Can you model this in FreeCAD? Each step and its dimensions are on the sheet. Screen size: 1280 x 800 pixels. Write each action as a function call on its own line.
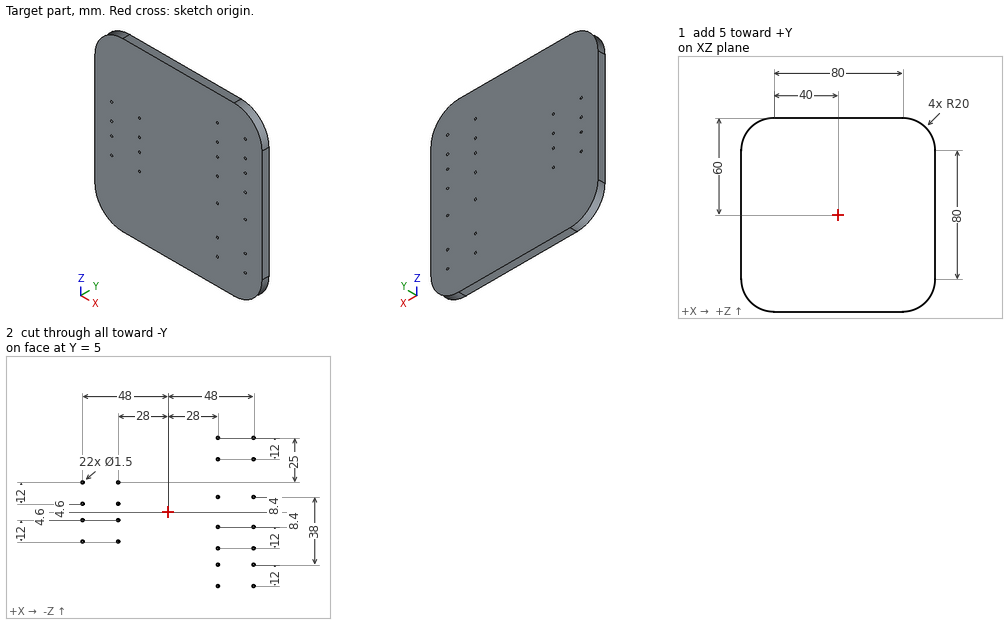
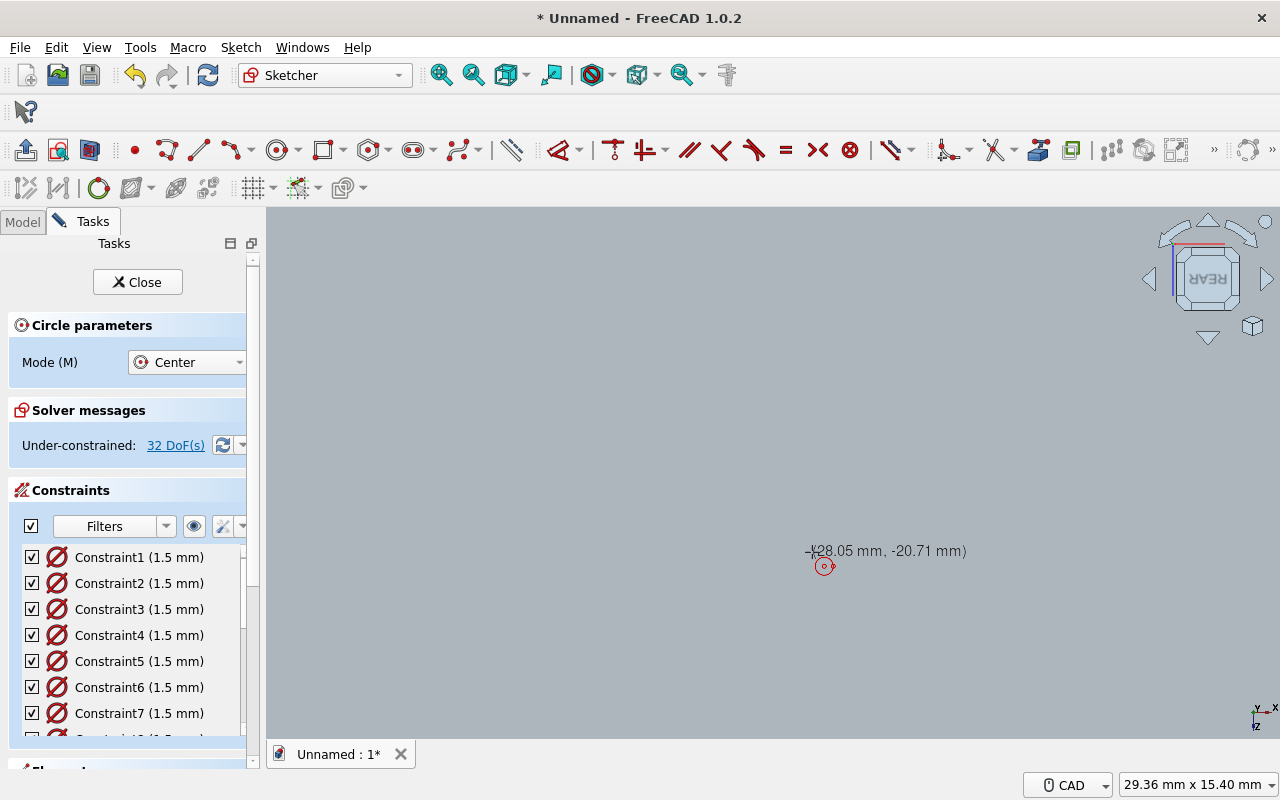
scroll(812, 552, down, 11)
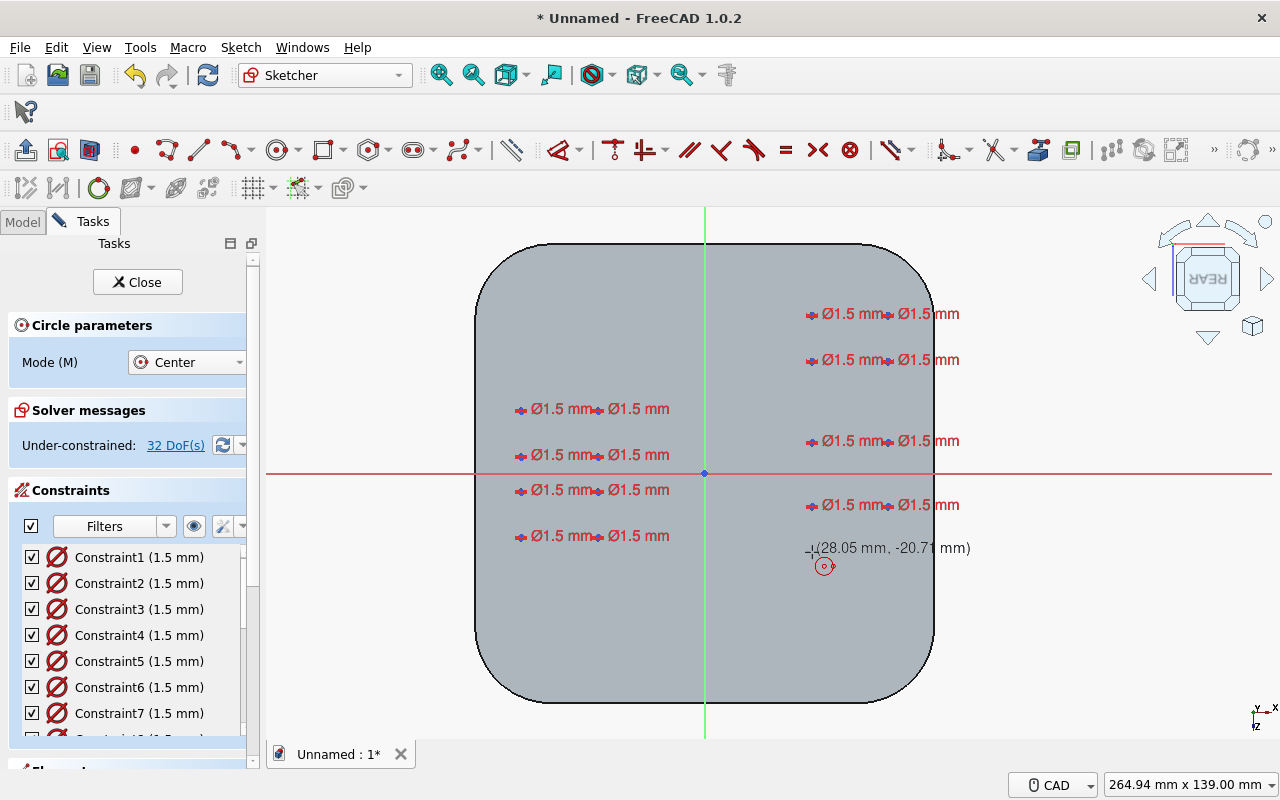
click(812, 552)
move(814, 550)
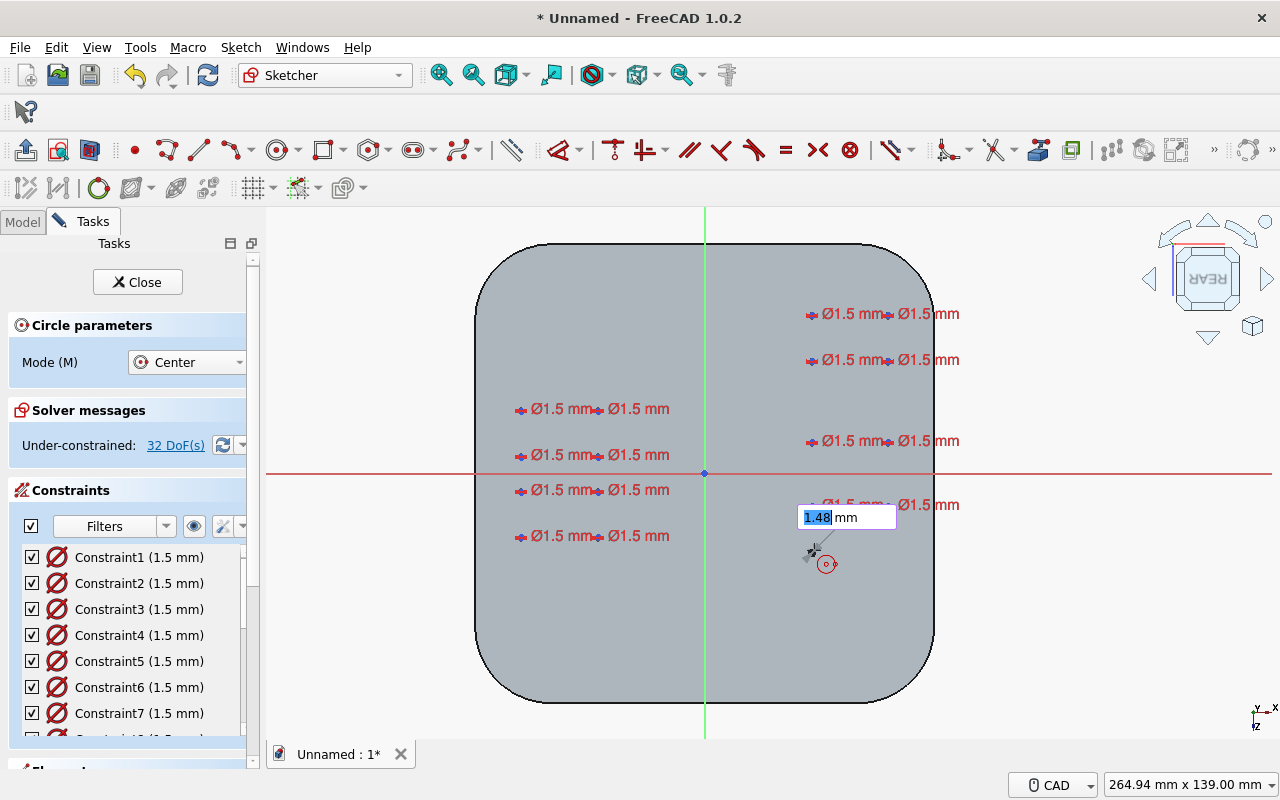
text(1.5)
key(Return)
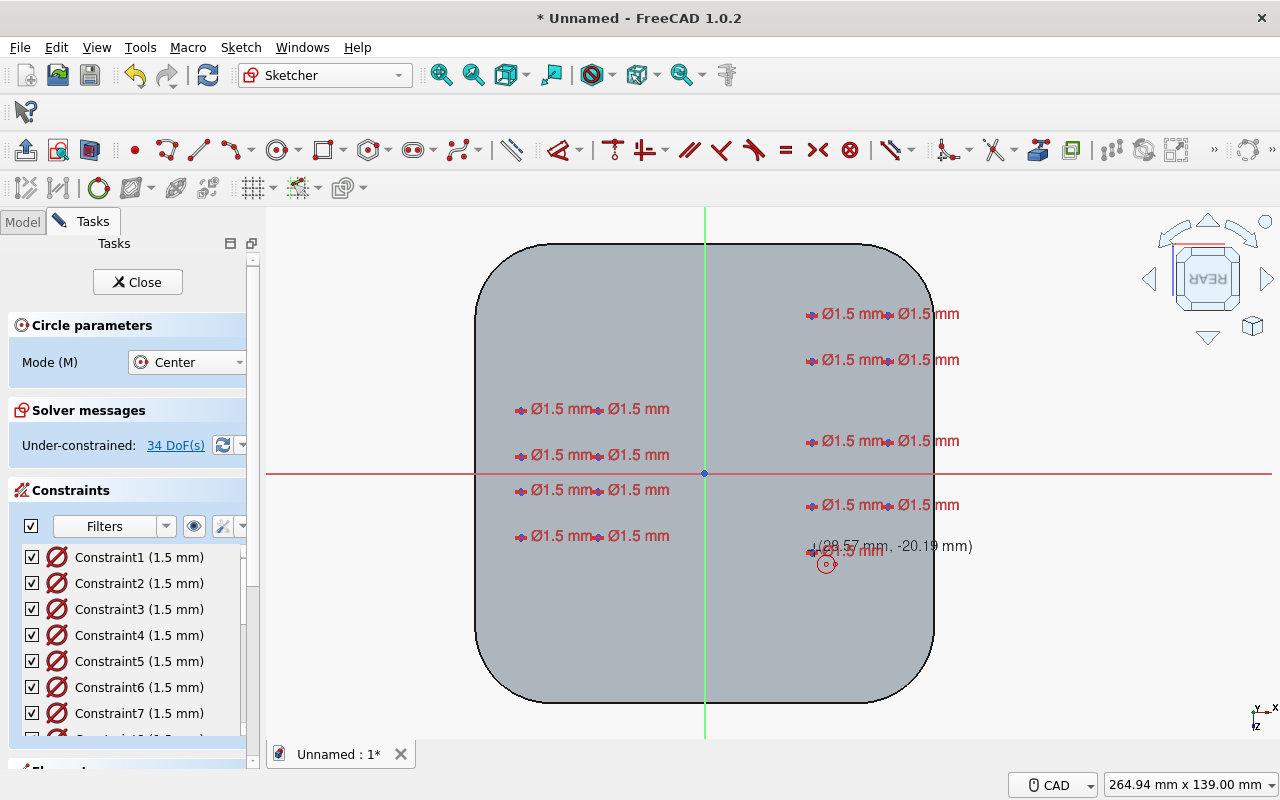
scroll(888, 552, up, 11)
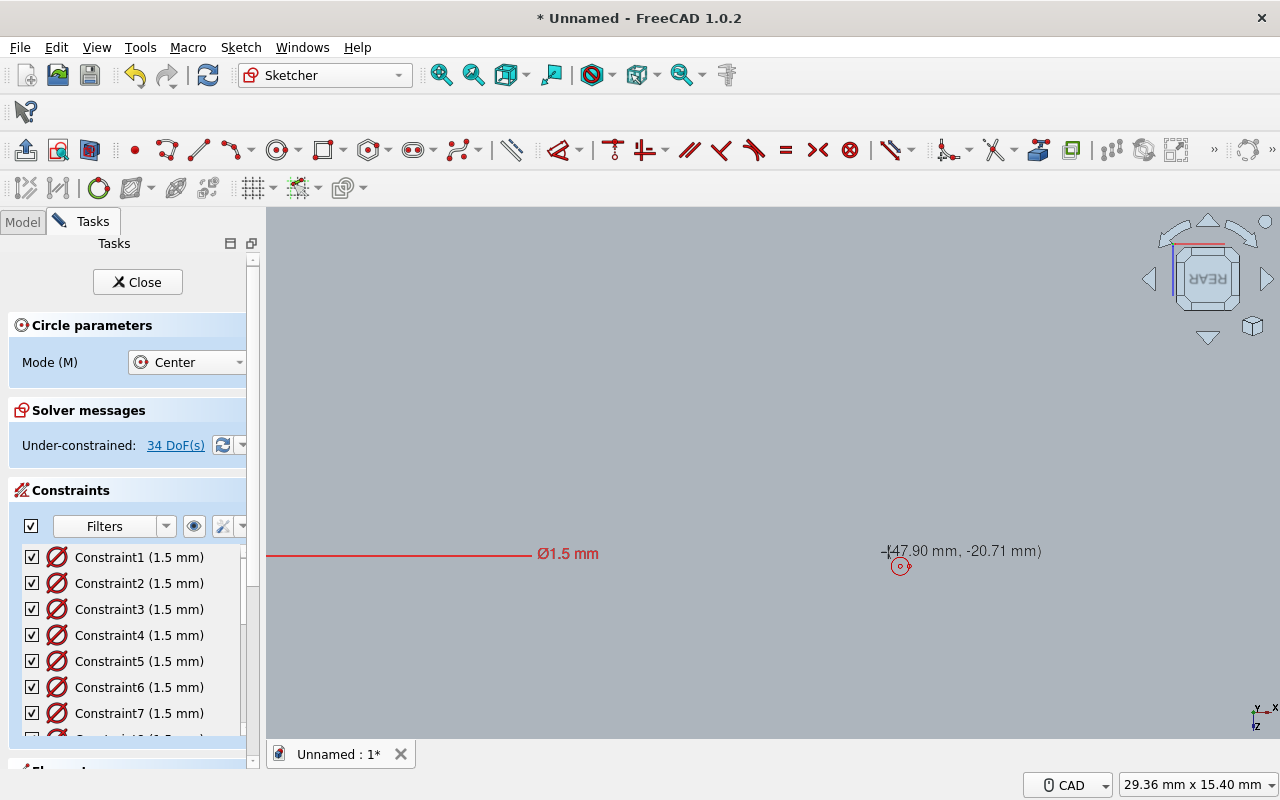
scroll(888, 552, down, 11)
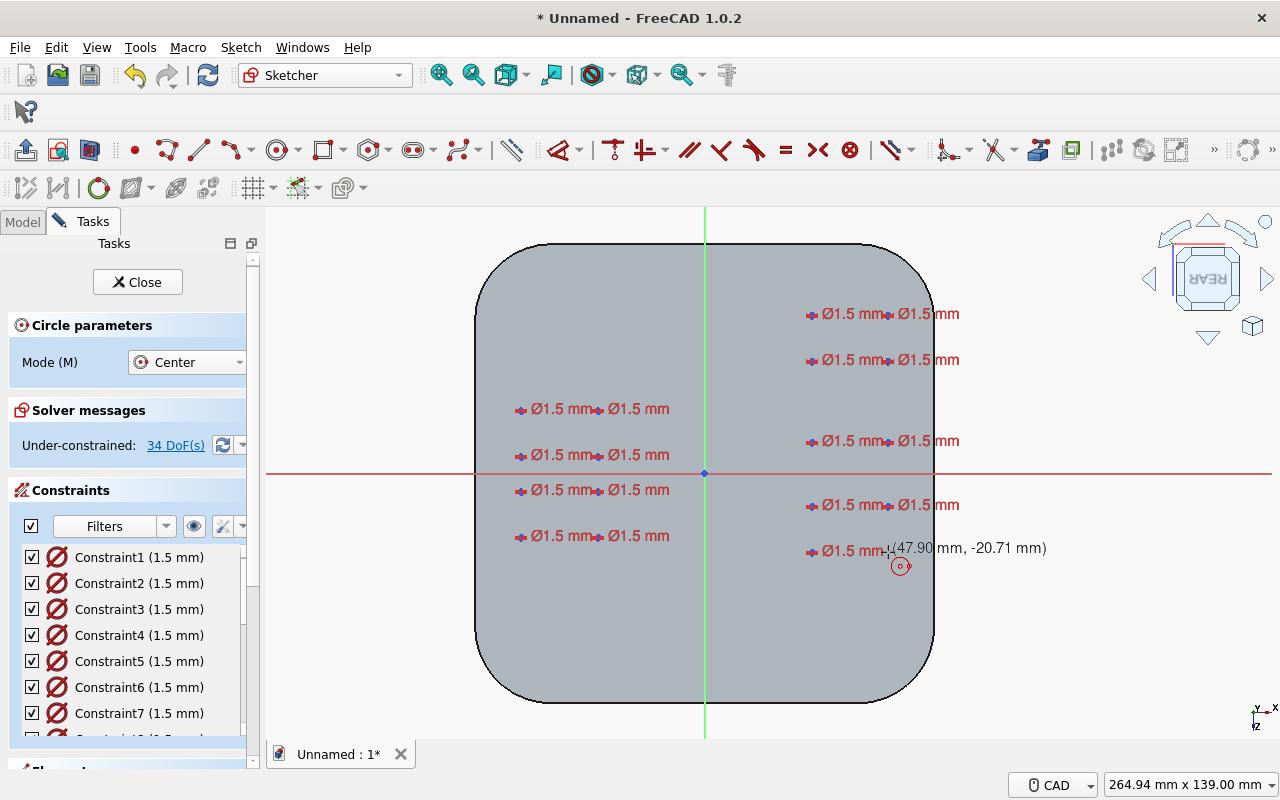
click(888, 552)
move(890, 550)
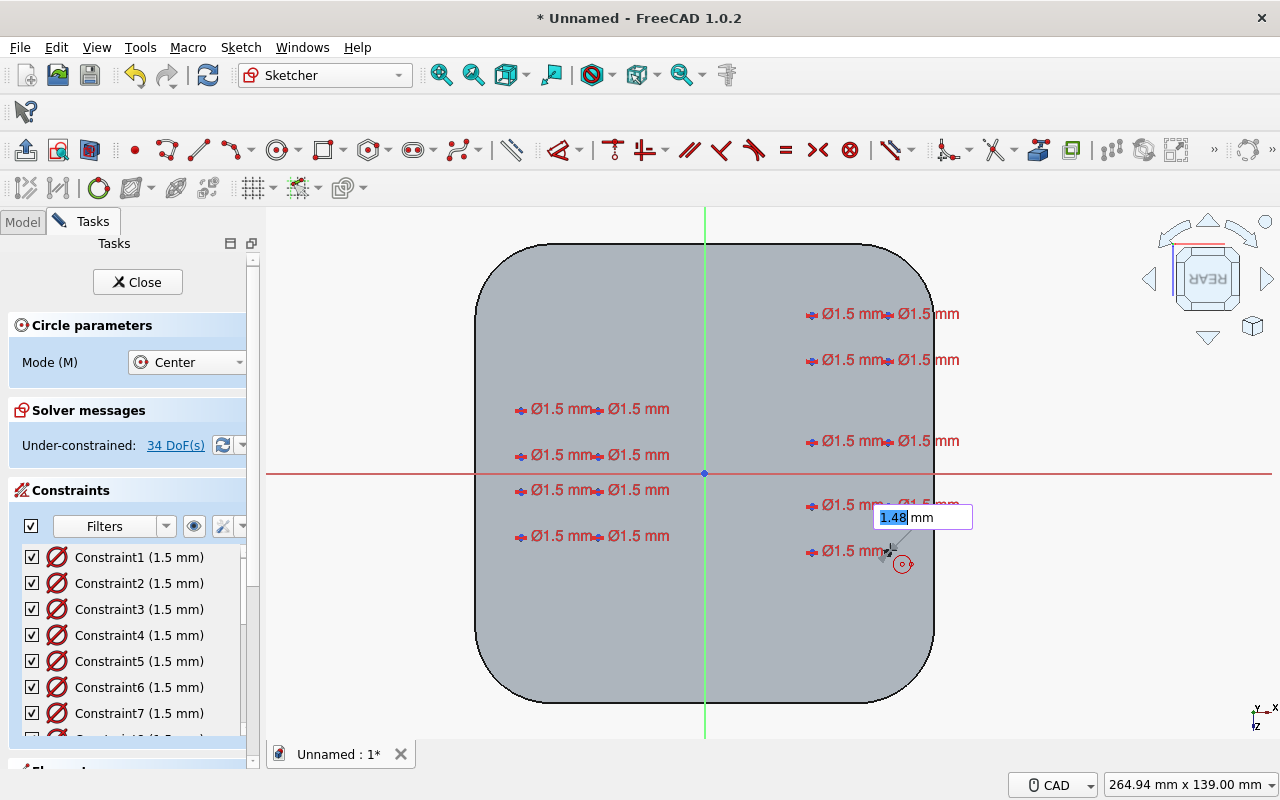
text(1.5)
key(Return)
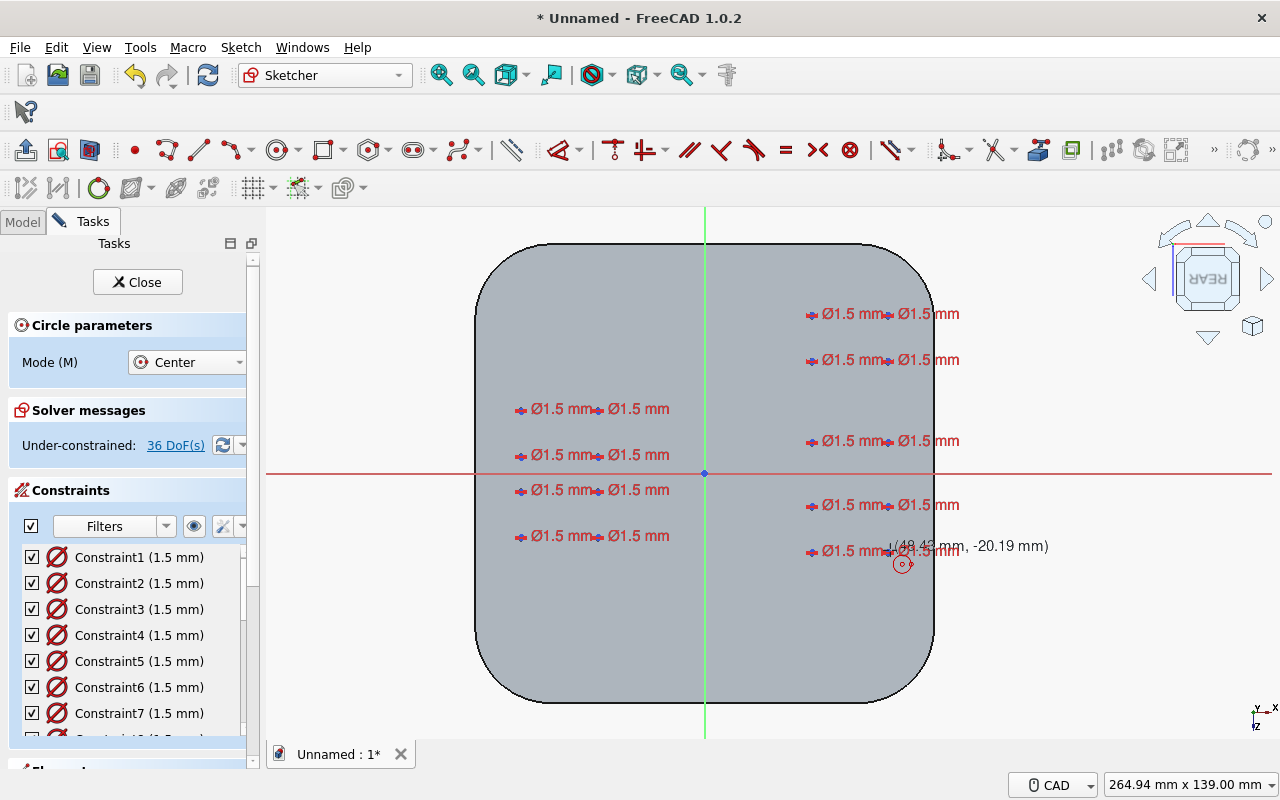
scroll(888, 587, up, 11)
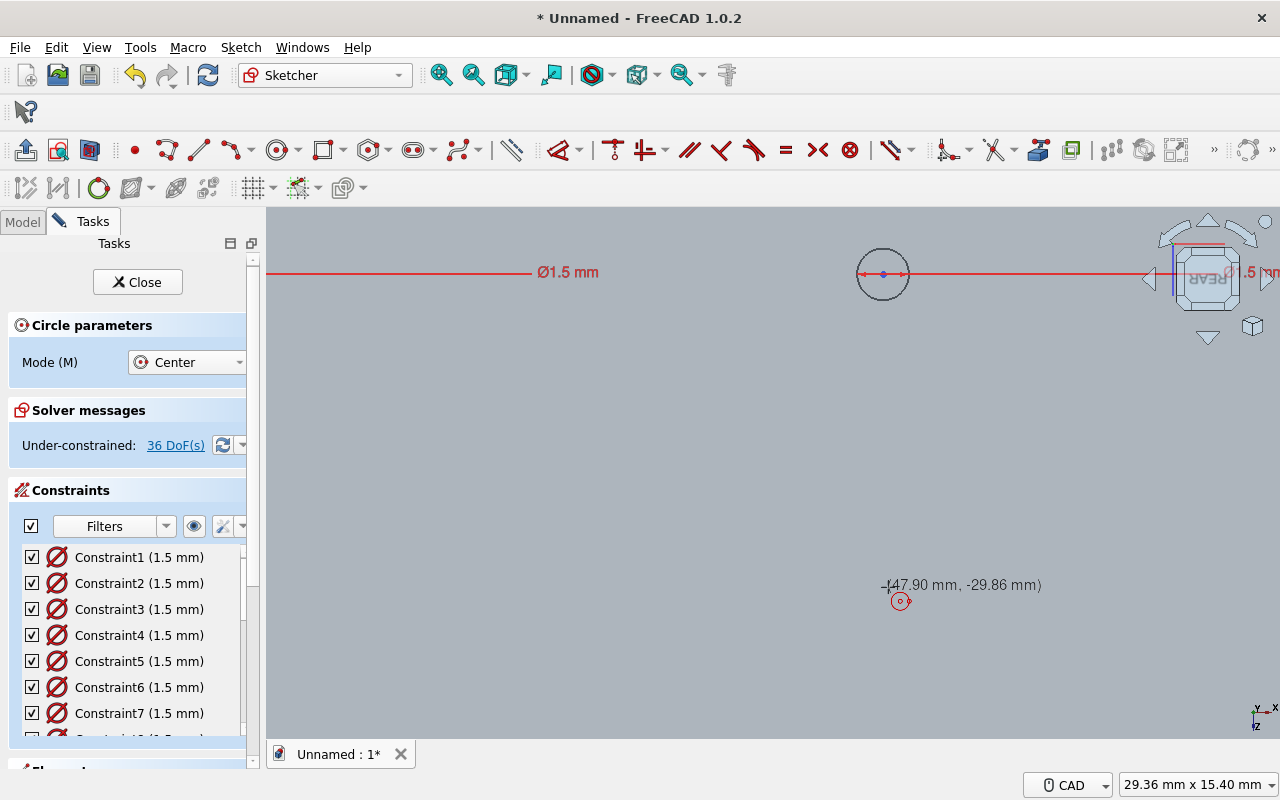
scroll(888, 587, down, 11)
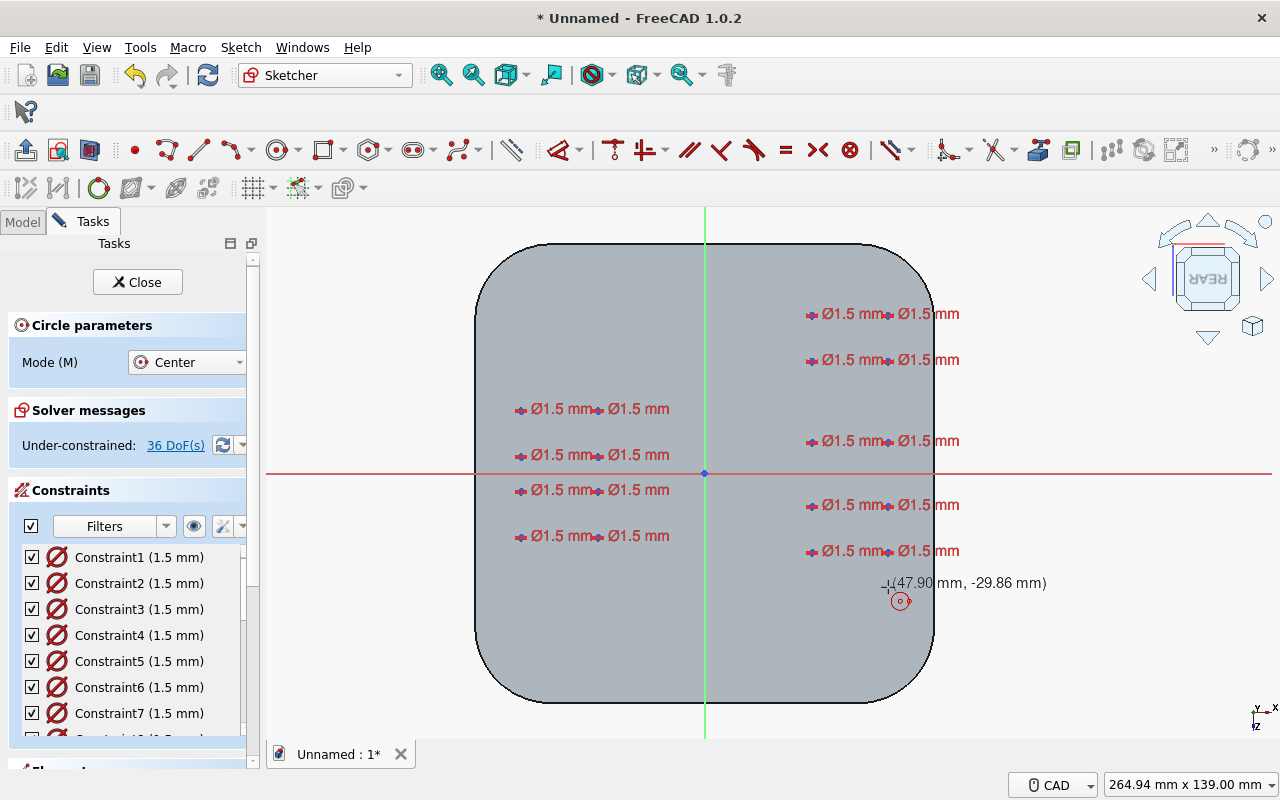
click(888, 587)
move(890, 585)